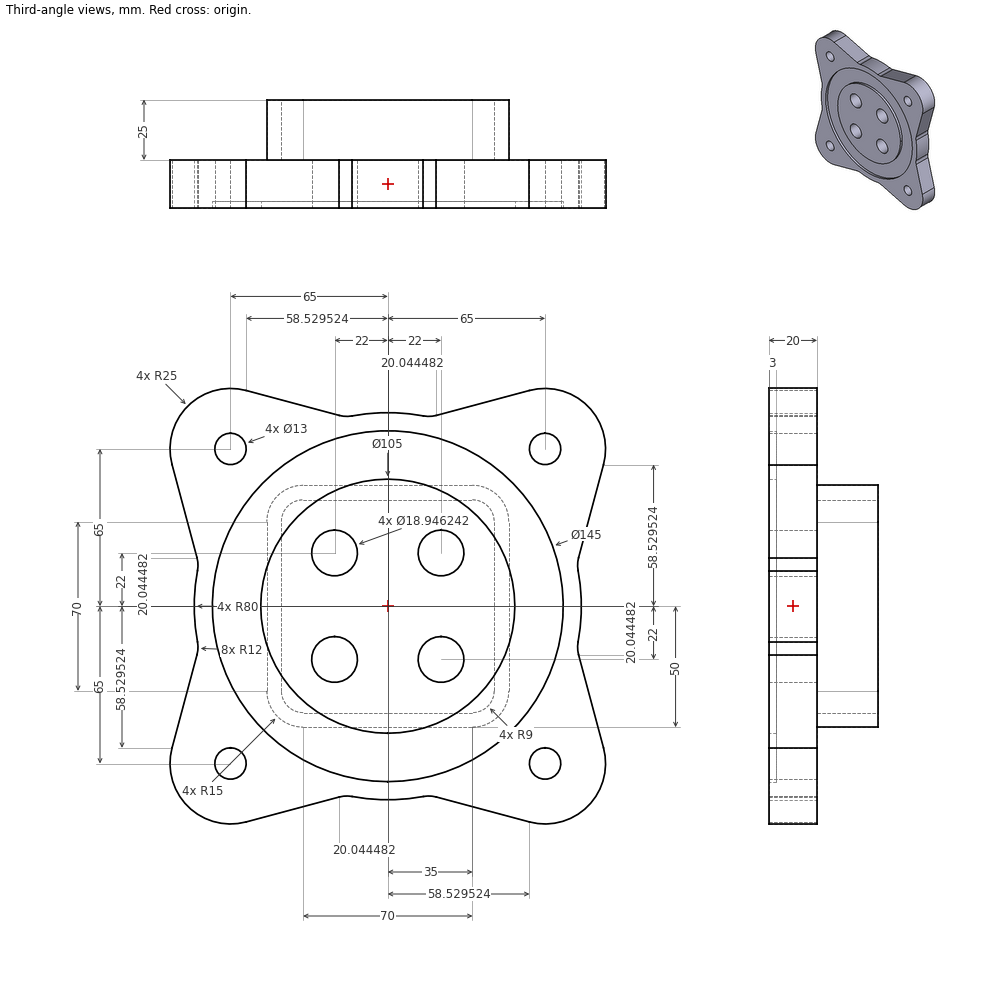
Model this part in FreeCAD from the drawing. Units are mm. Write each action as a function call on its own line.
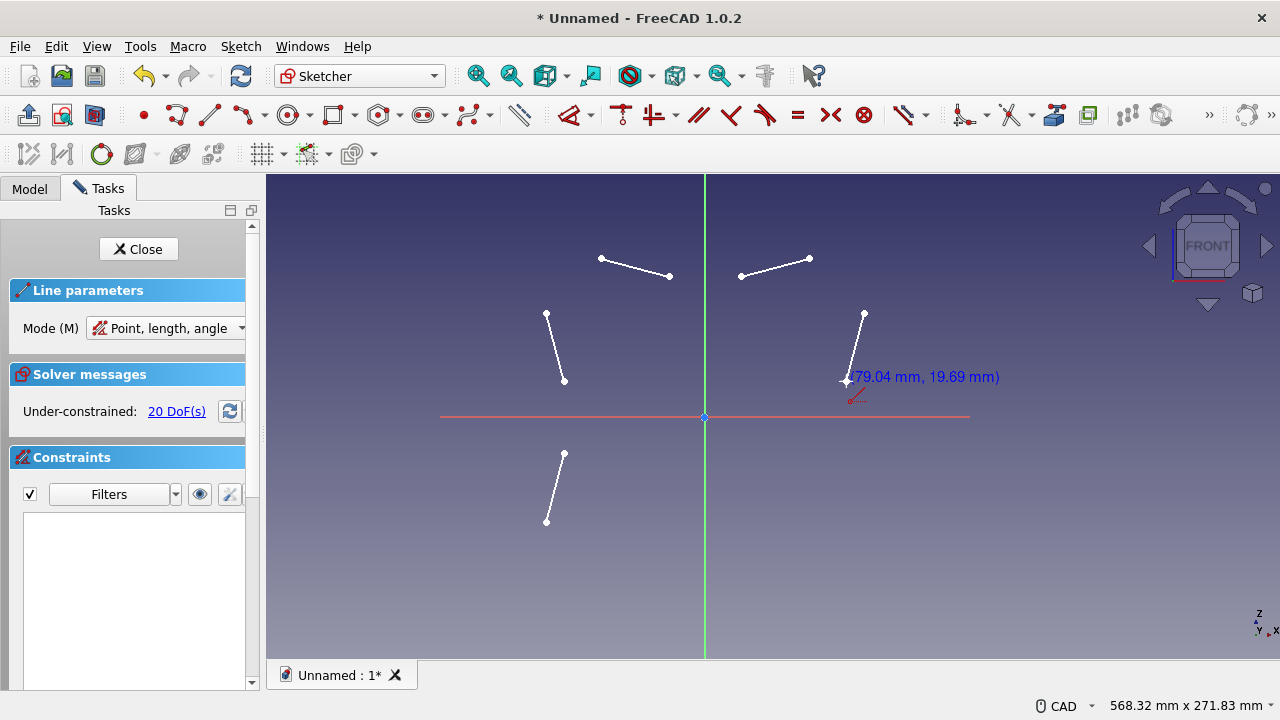
click(846, 453)
click(864, 522)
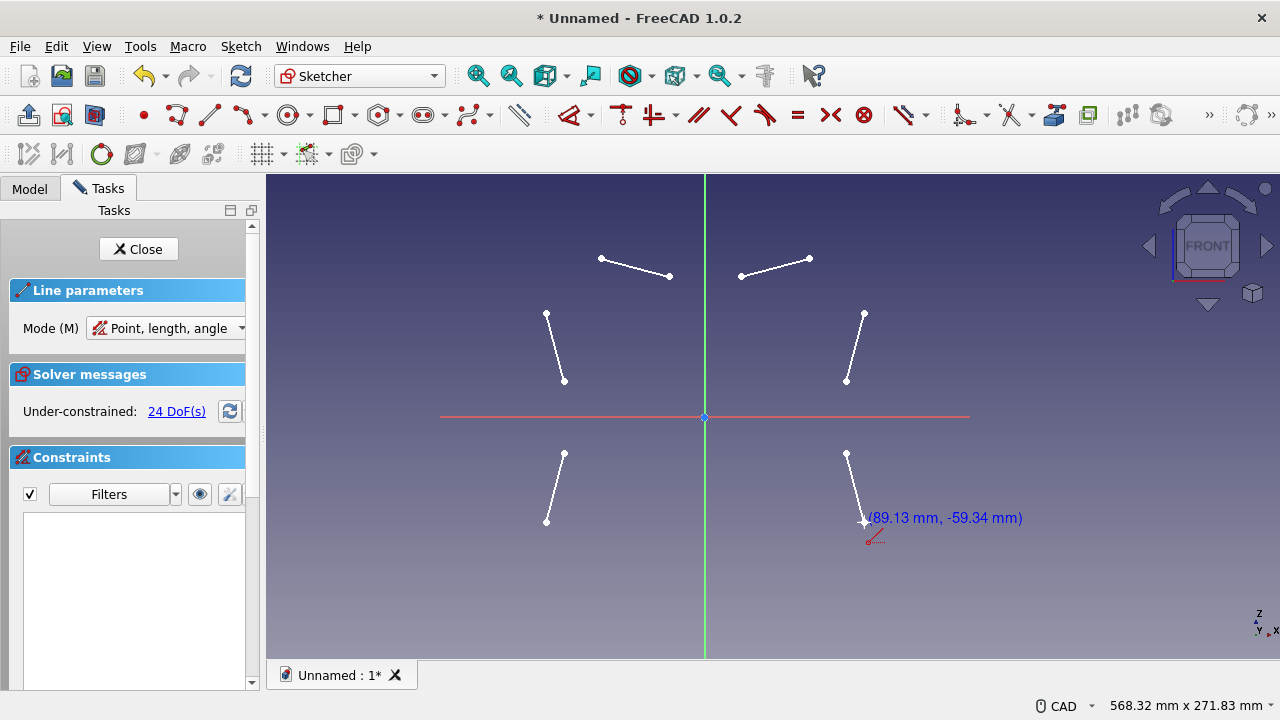
click(809, 576)
click(741, 558)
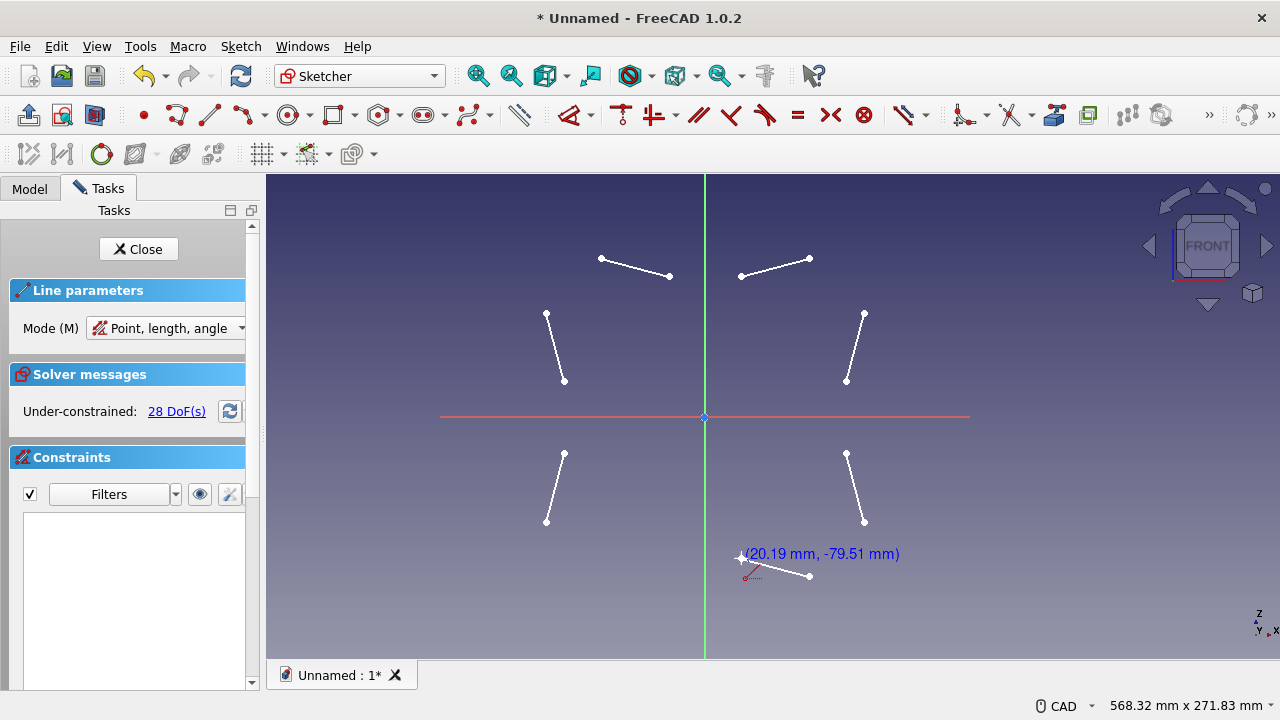
click(669, 558)
click(601, 576)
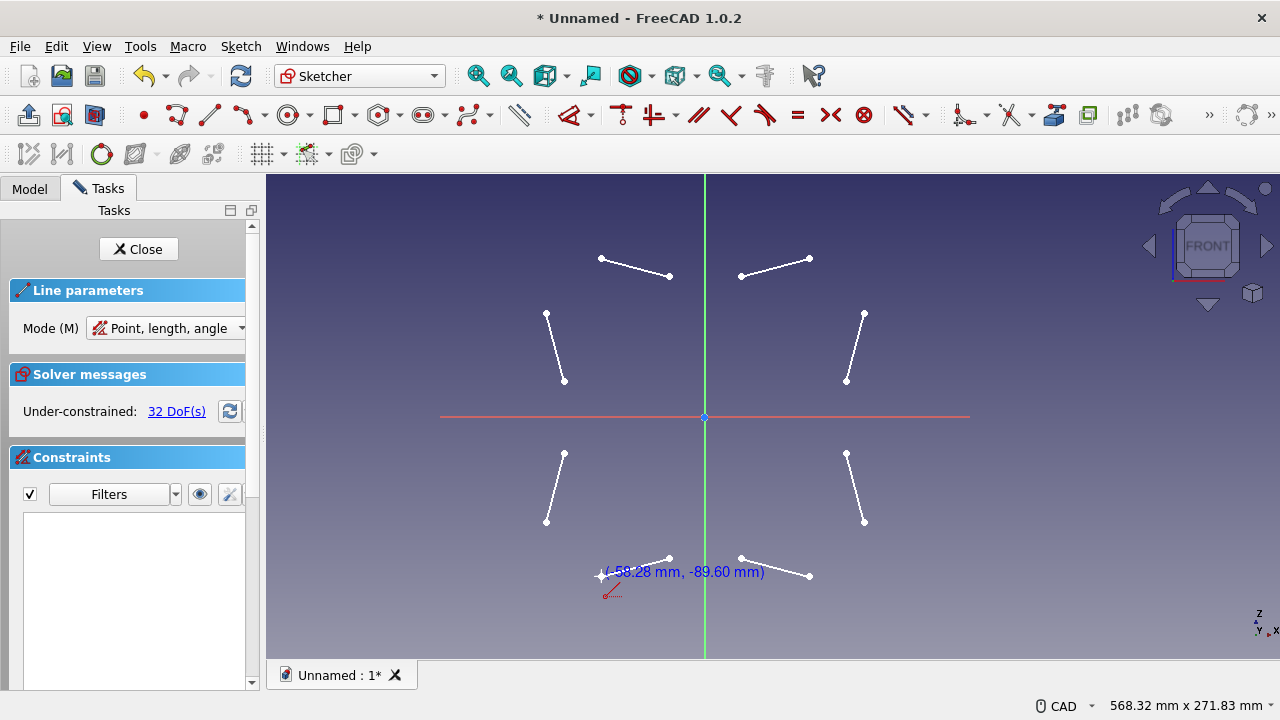
click(242, 116)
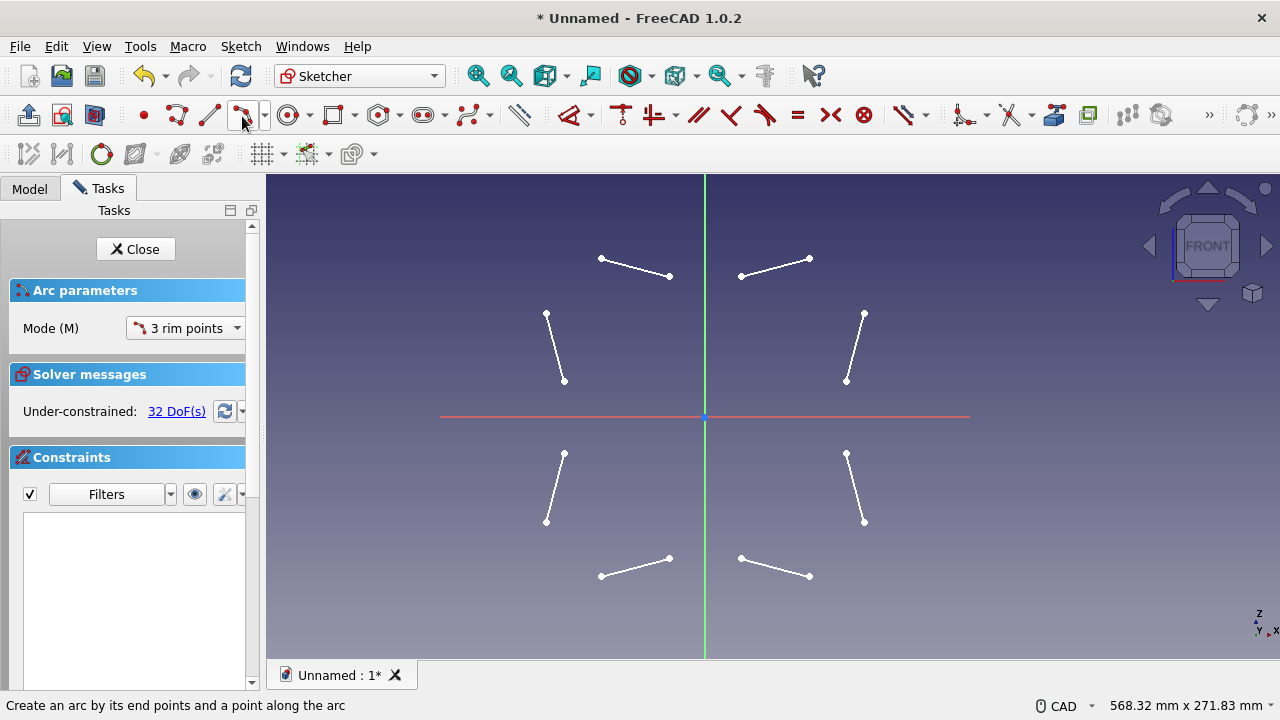
click(564, 454)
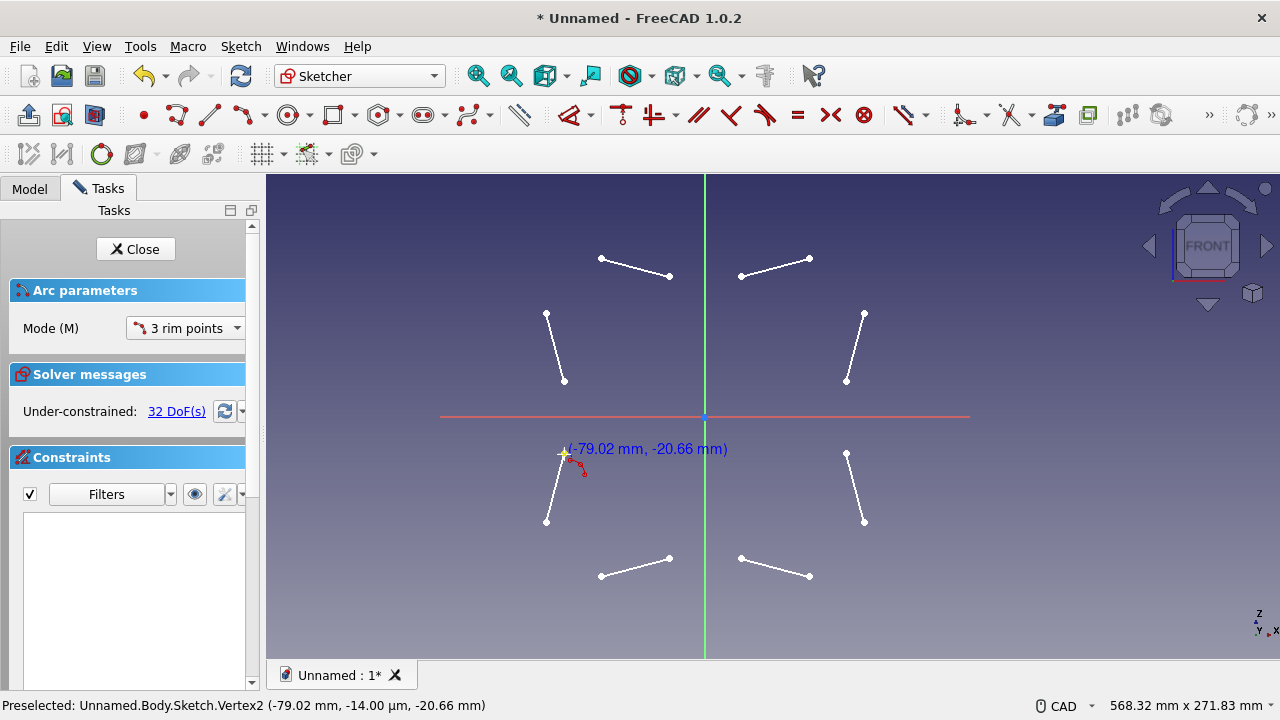
scroll(565, 443, up, 3)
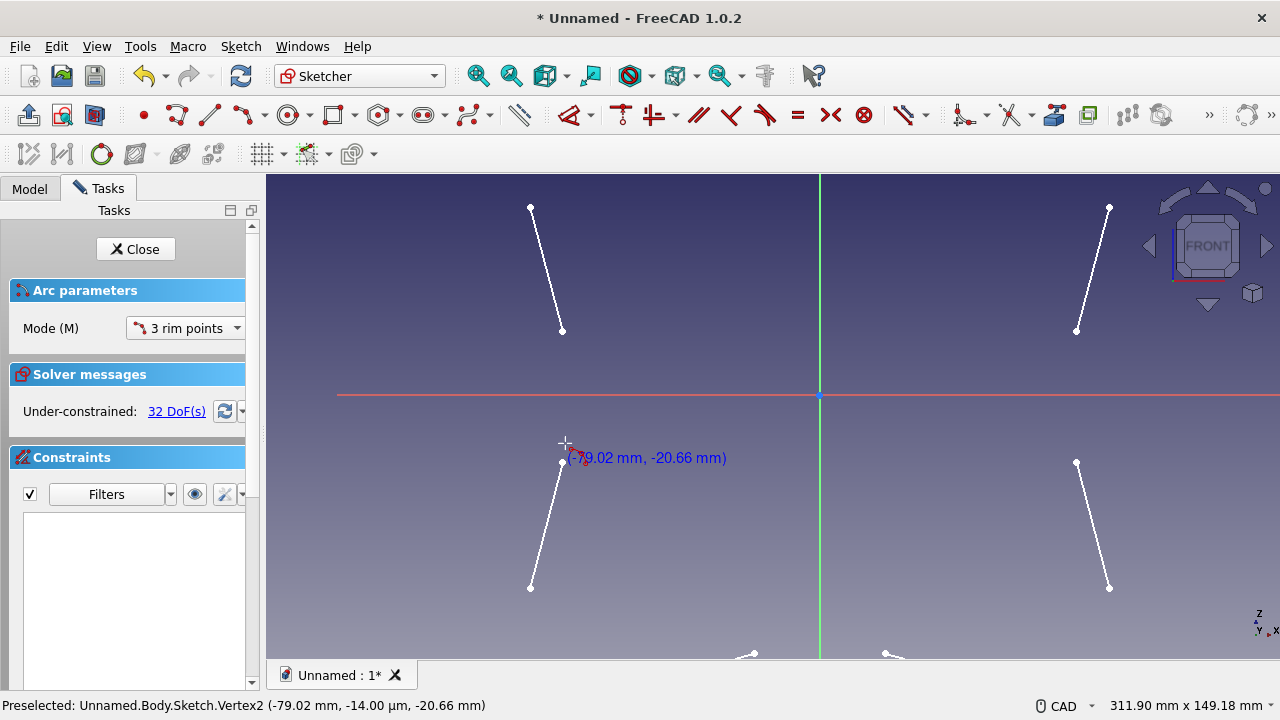
click(564, 443)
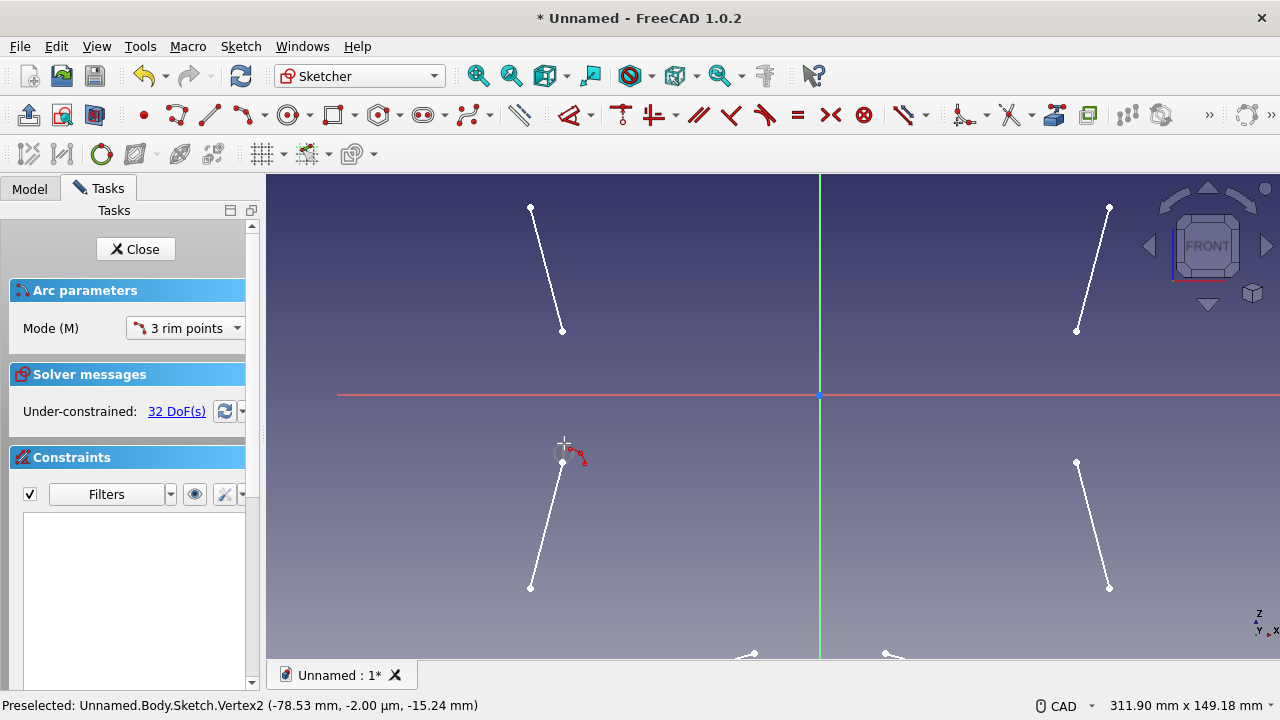
scroll(565, 452, up, 14)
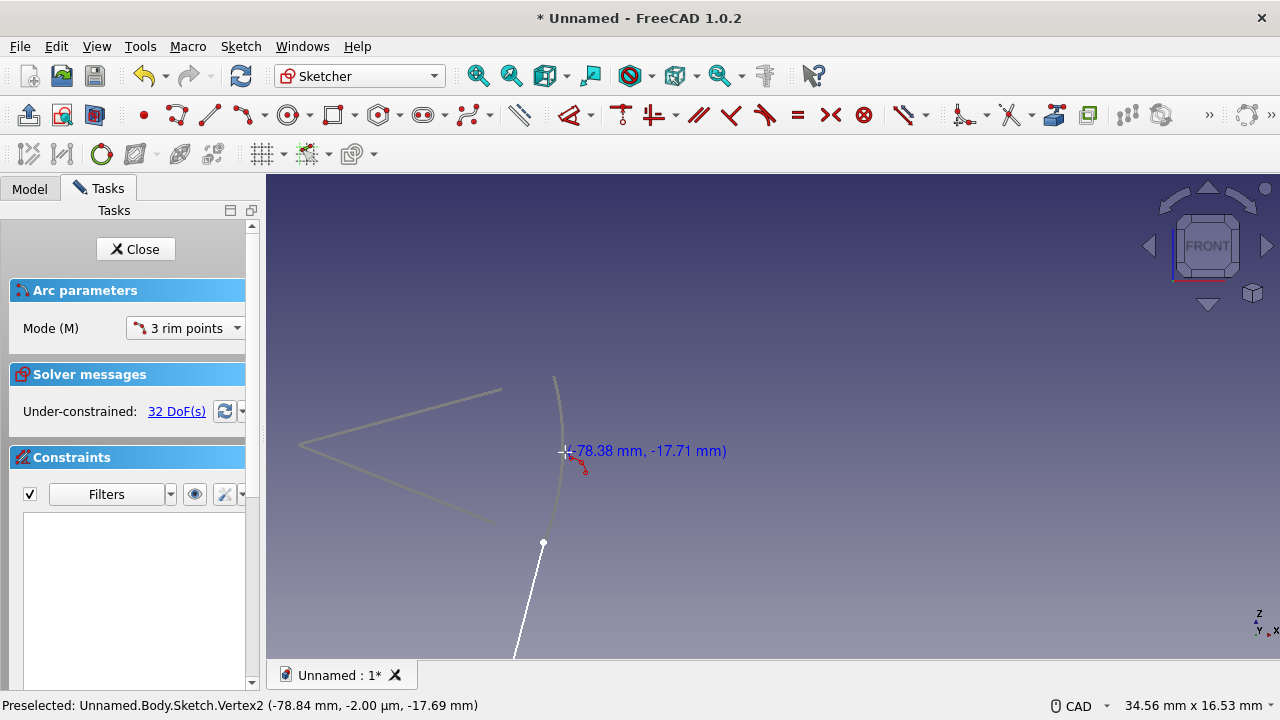
click(557, 443)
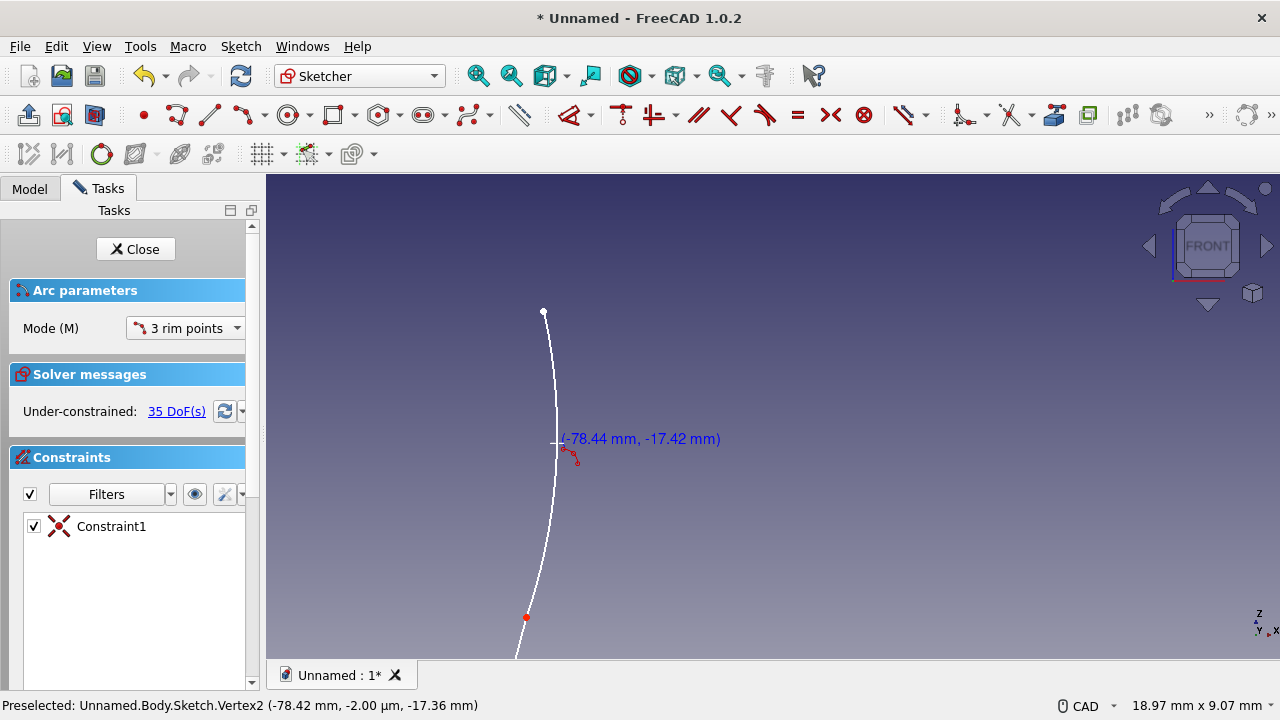
scroll(565, 448, down, 17)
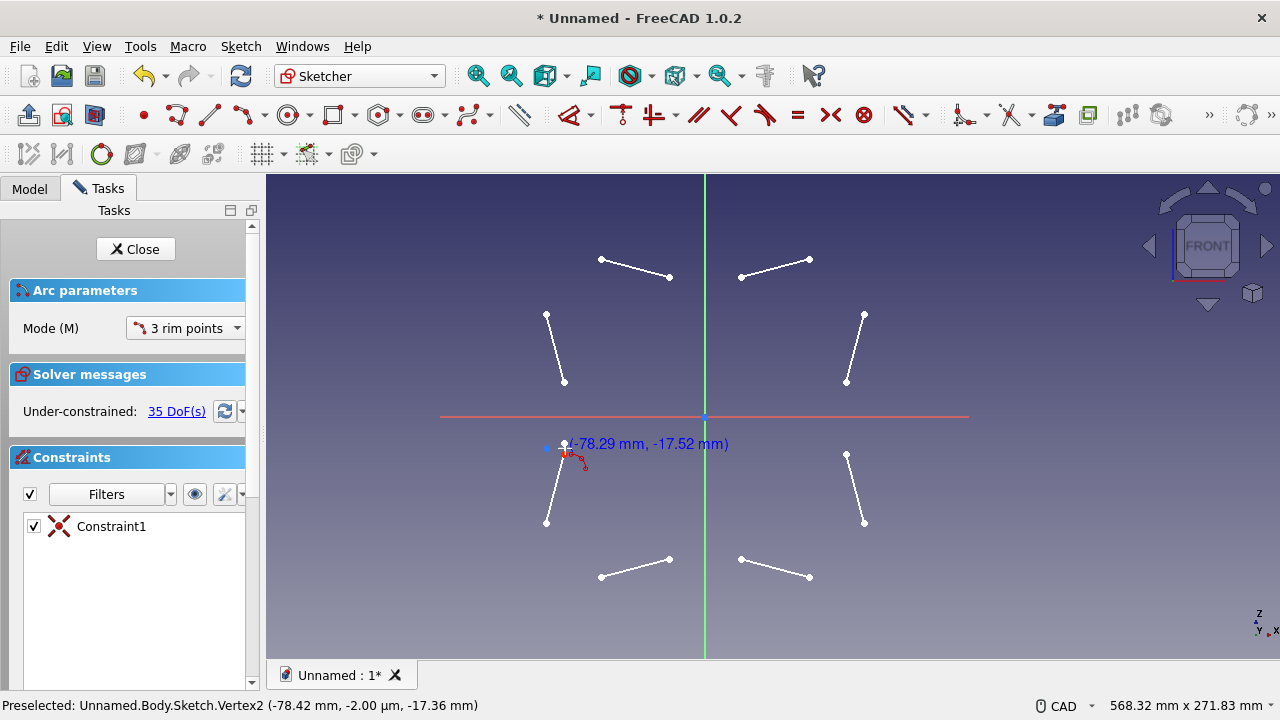
scroll(565, 444, up, 3)